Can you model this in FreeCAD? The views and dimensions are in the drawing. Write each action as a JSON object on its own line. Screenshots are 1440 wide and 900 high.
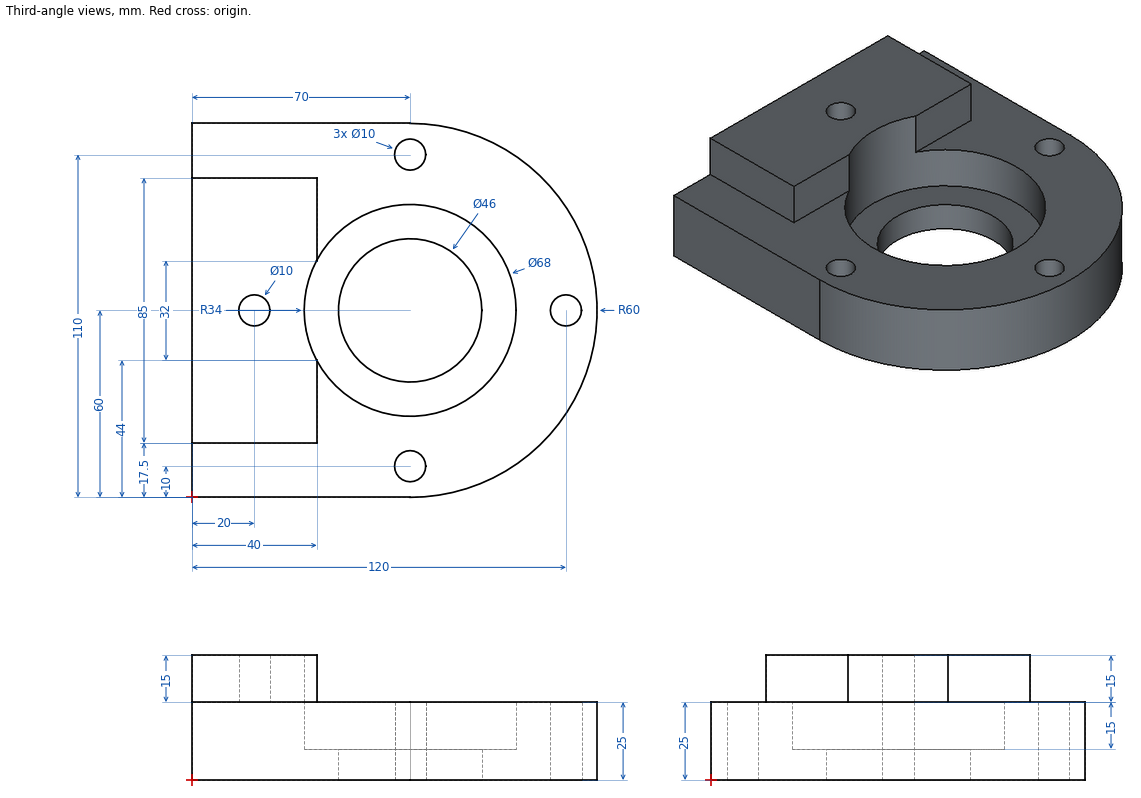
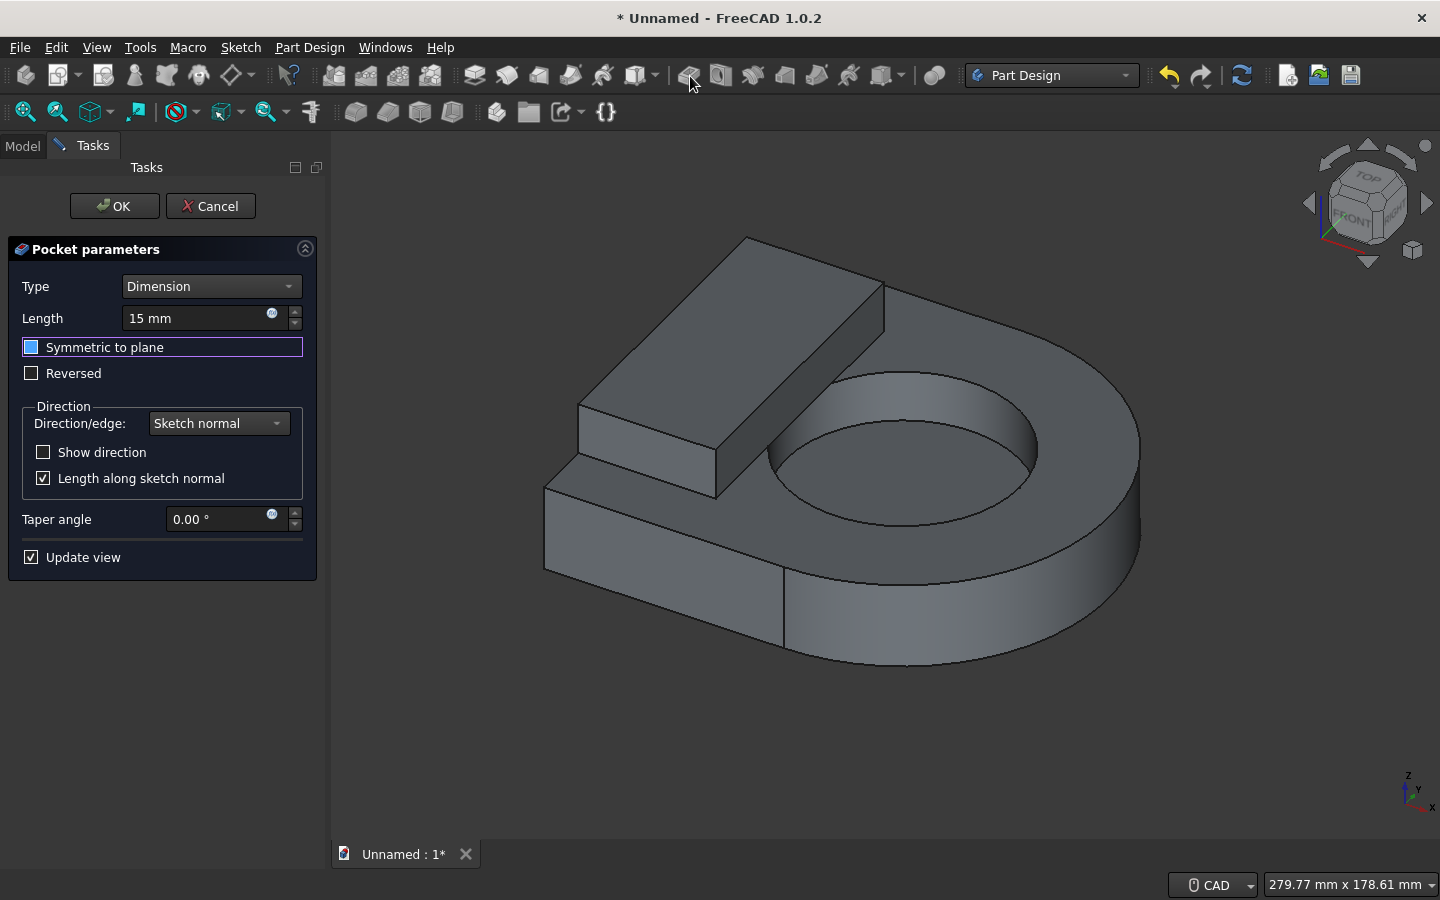
{"action": "left_click", "coordinate": [115, 206]}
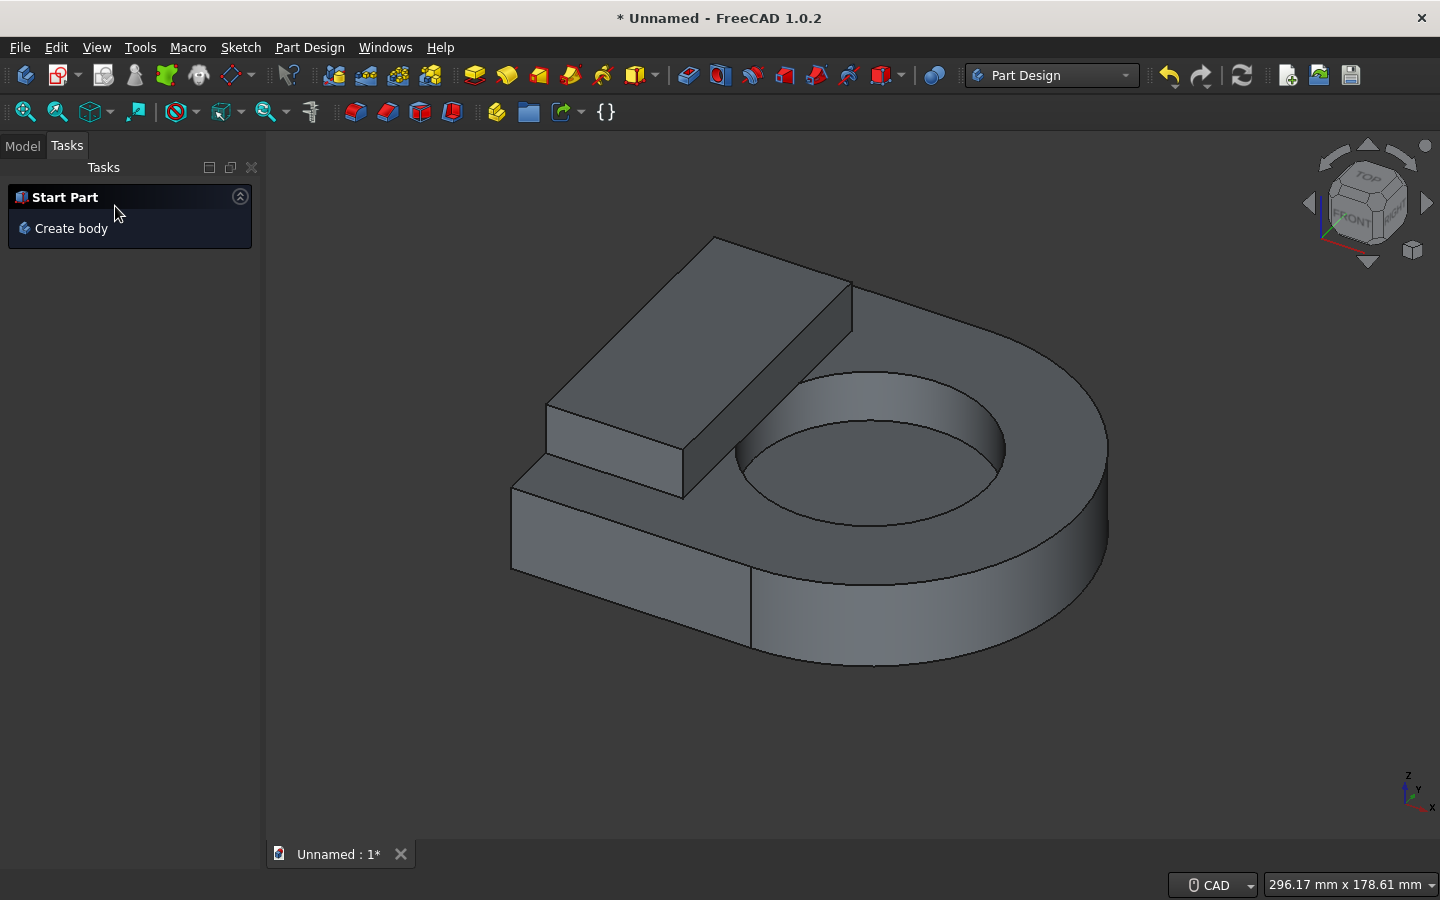
{"action": "left_click", "coordinate": [723, 318]}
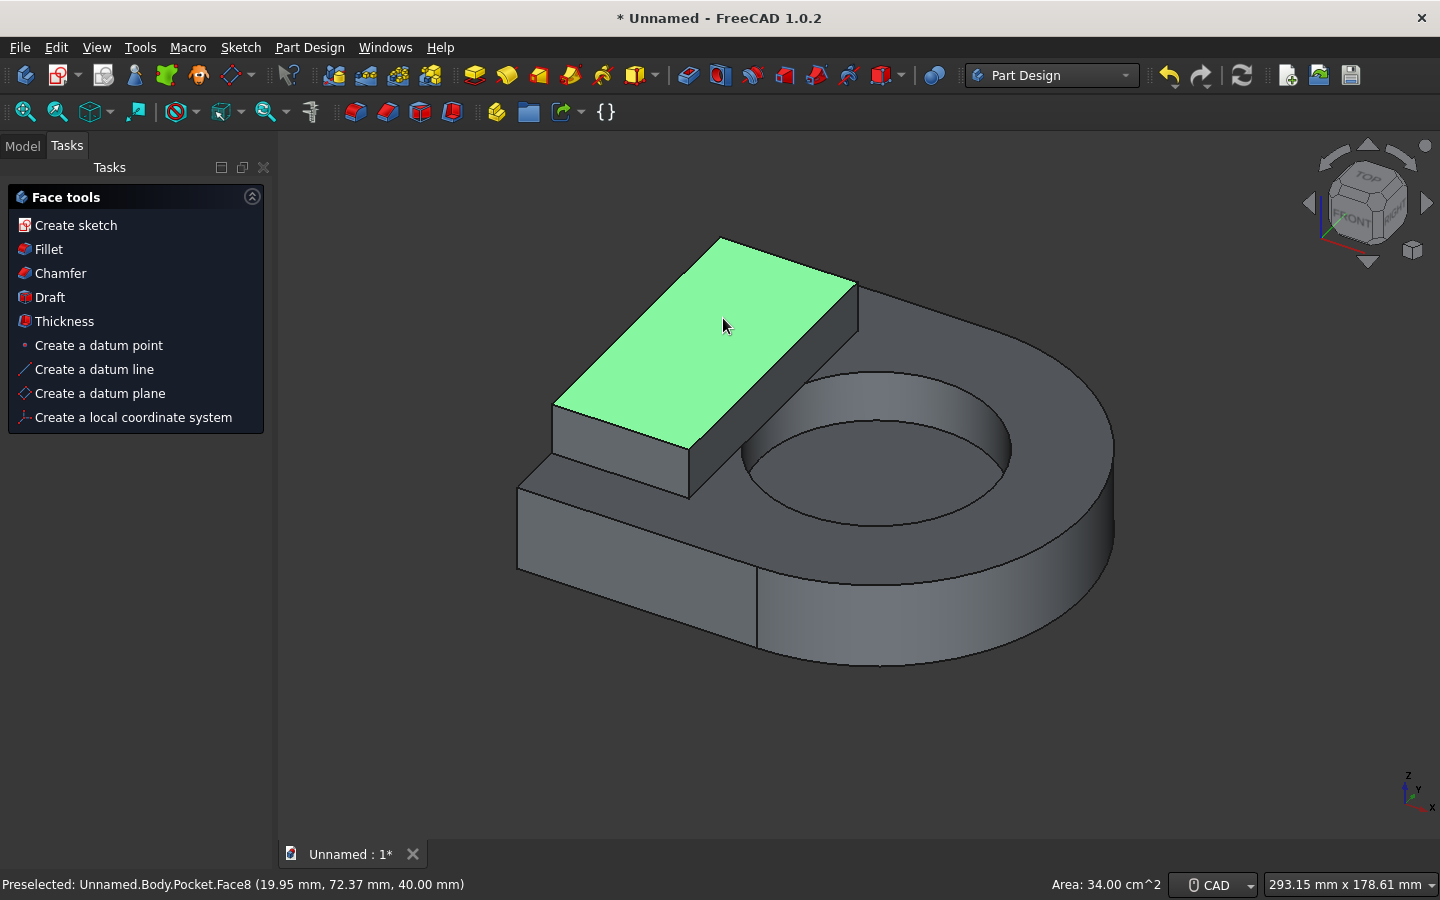
{"action": "left_click", "coordinate": [58, 76]}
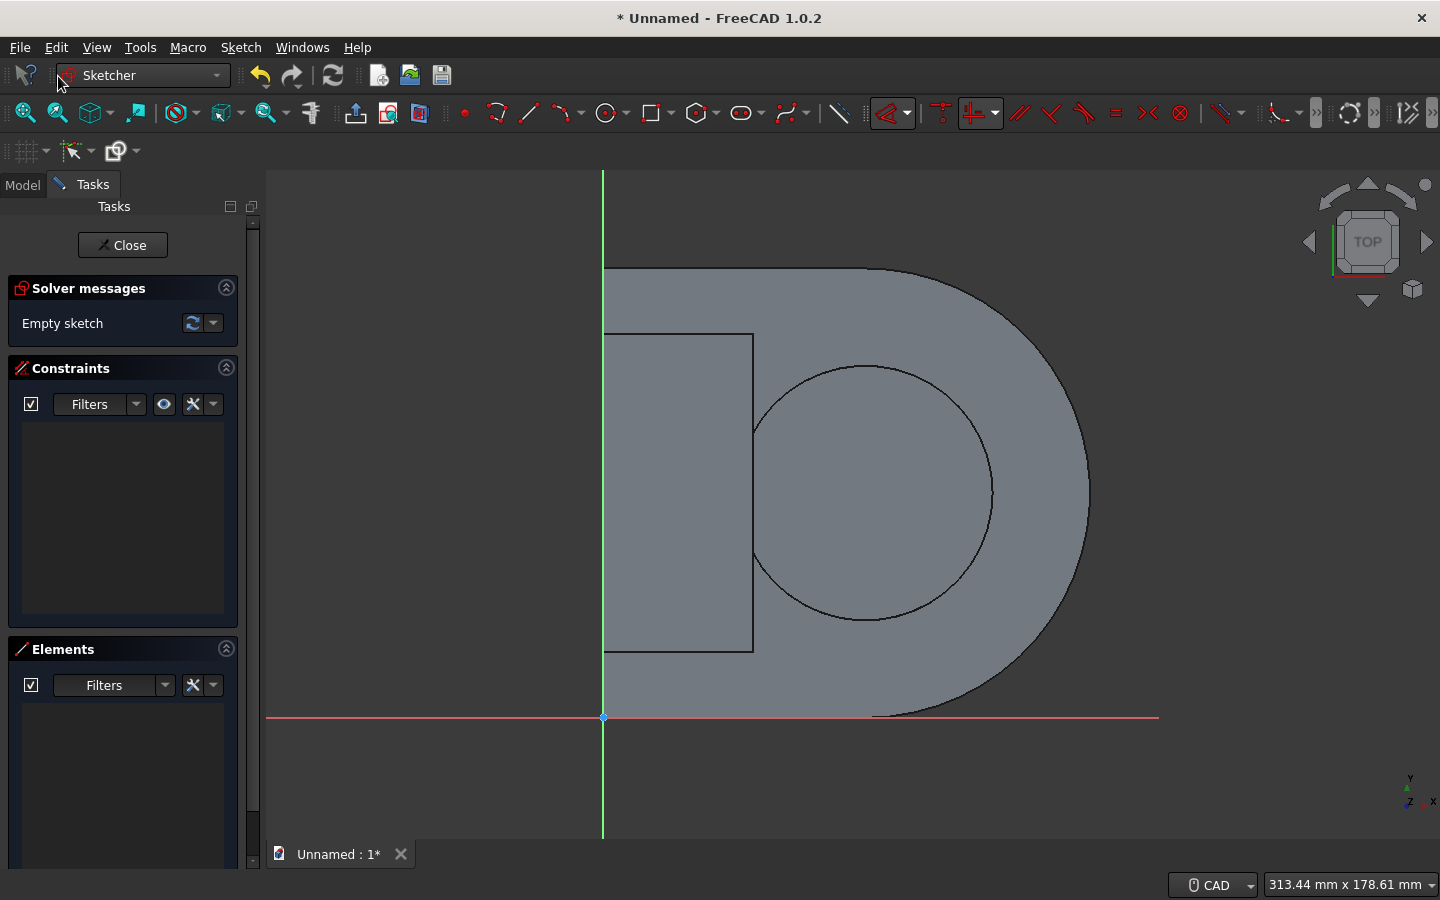
{"action": "scroll", "coordinate": [462, 720], "scroll_direction": "up", "scroll_amount": 2}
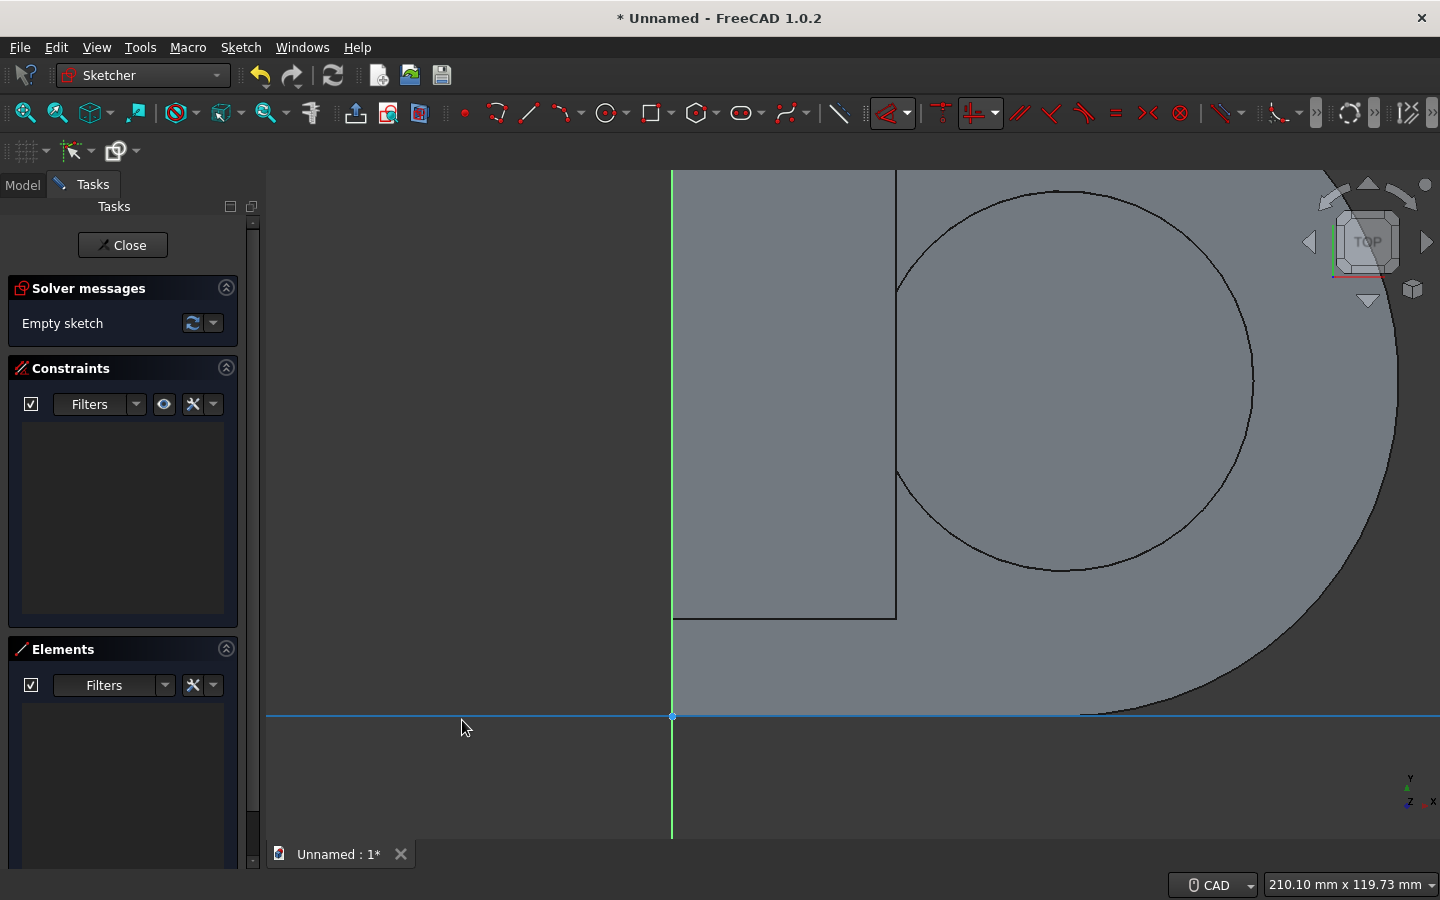
{"action": "left_click", "coordinate": [530, 114]}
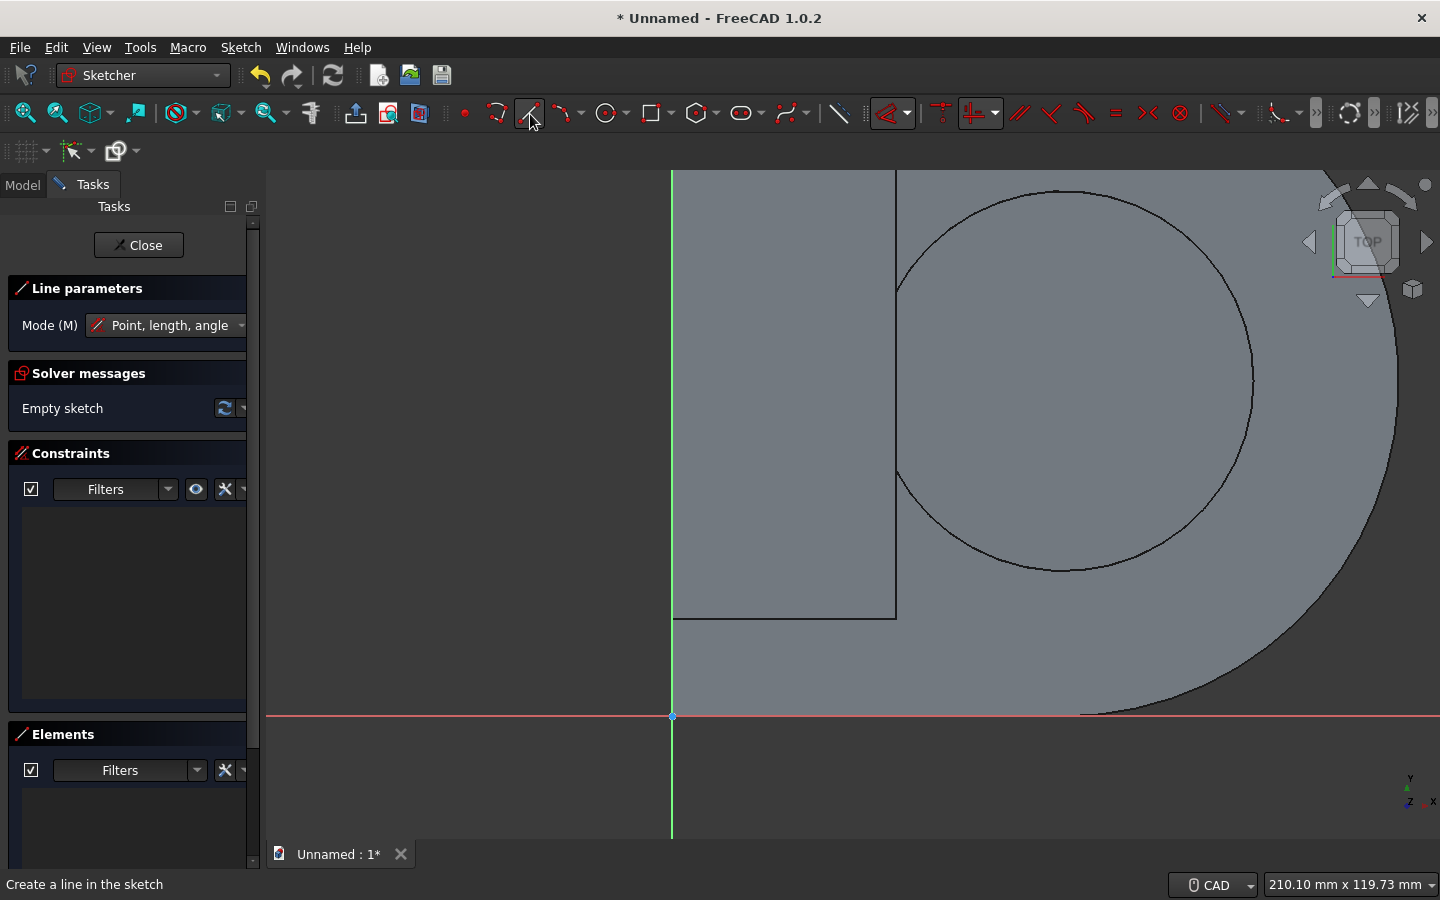
{"action": "left_click", "coordinate": [896, 471]}
{"action": "left_click", "coordinate": [896, 292]}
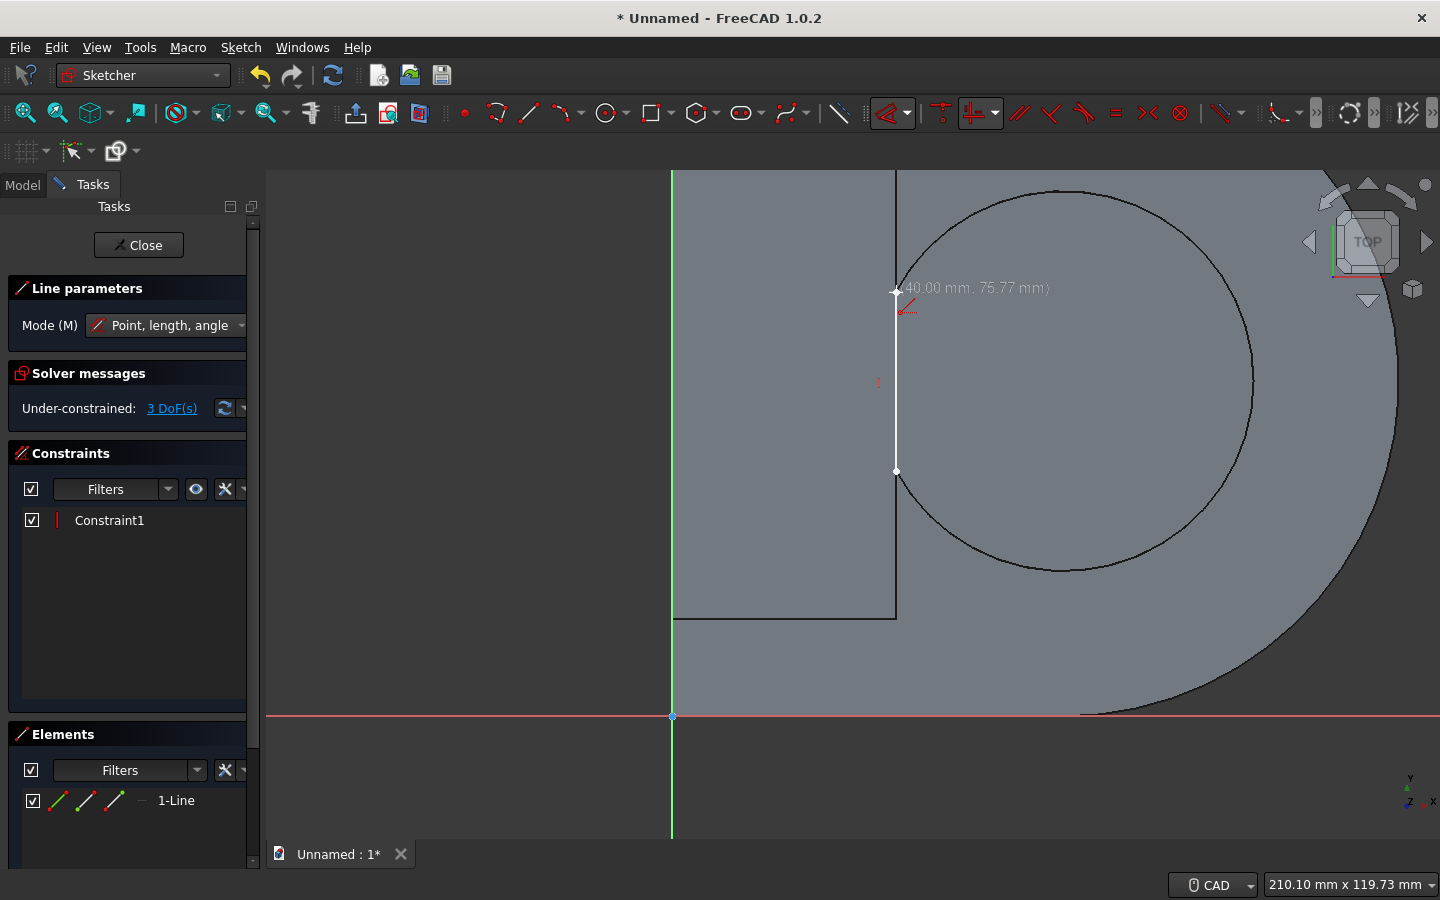
{"action": "left_click", "coordinate": [562, 114]}